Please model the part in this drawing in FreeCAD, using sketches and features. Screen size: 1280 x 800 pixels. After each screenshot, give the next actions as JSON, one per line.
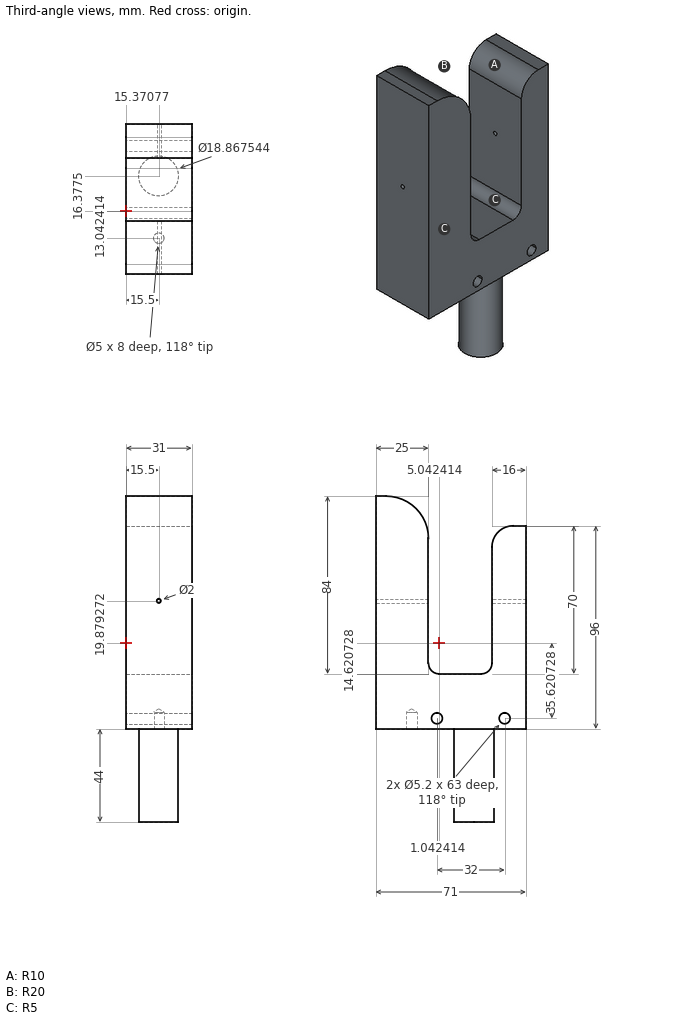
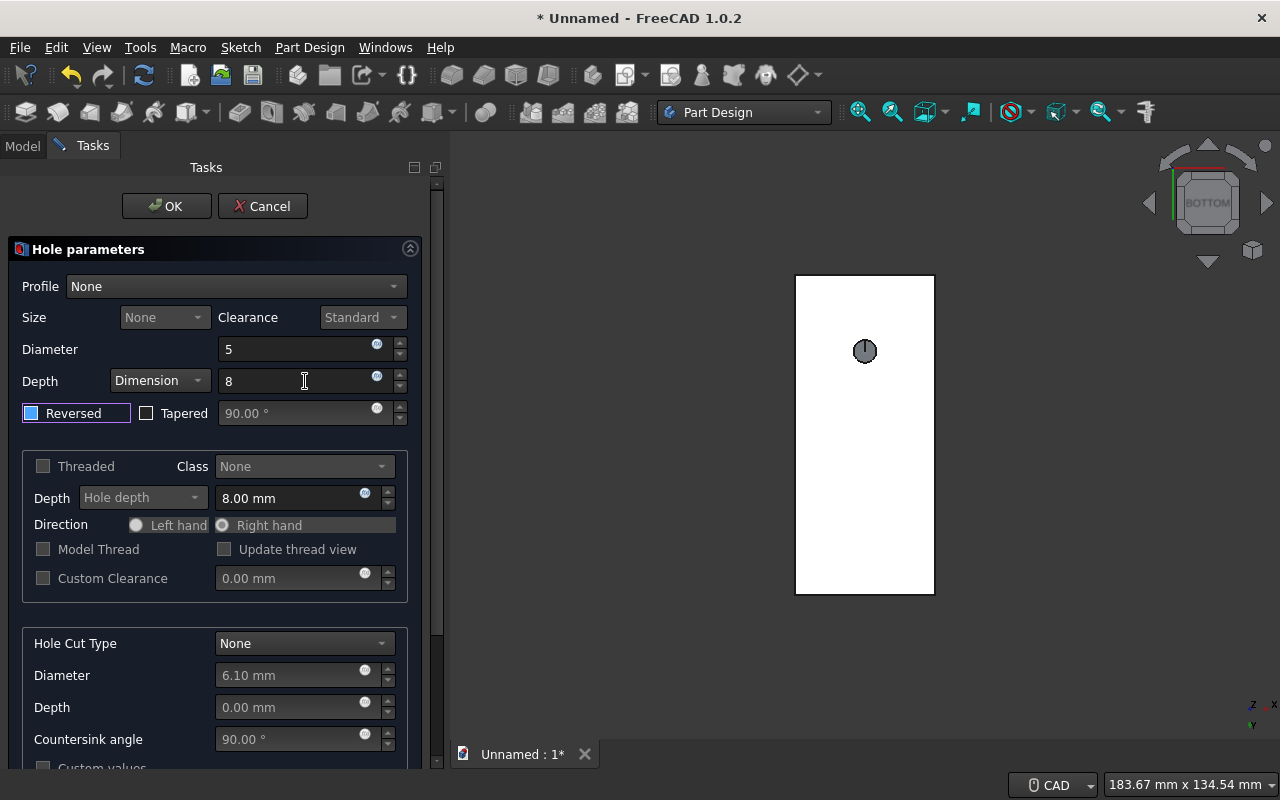
{"action": "left_click", "coordinate": [167, 206]}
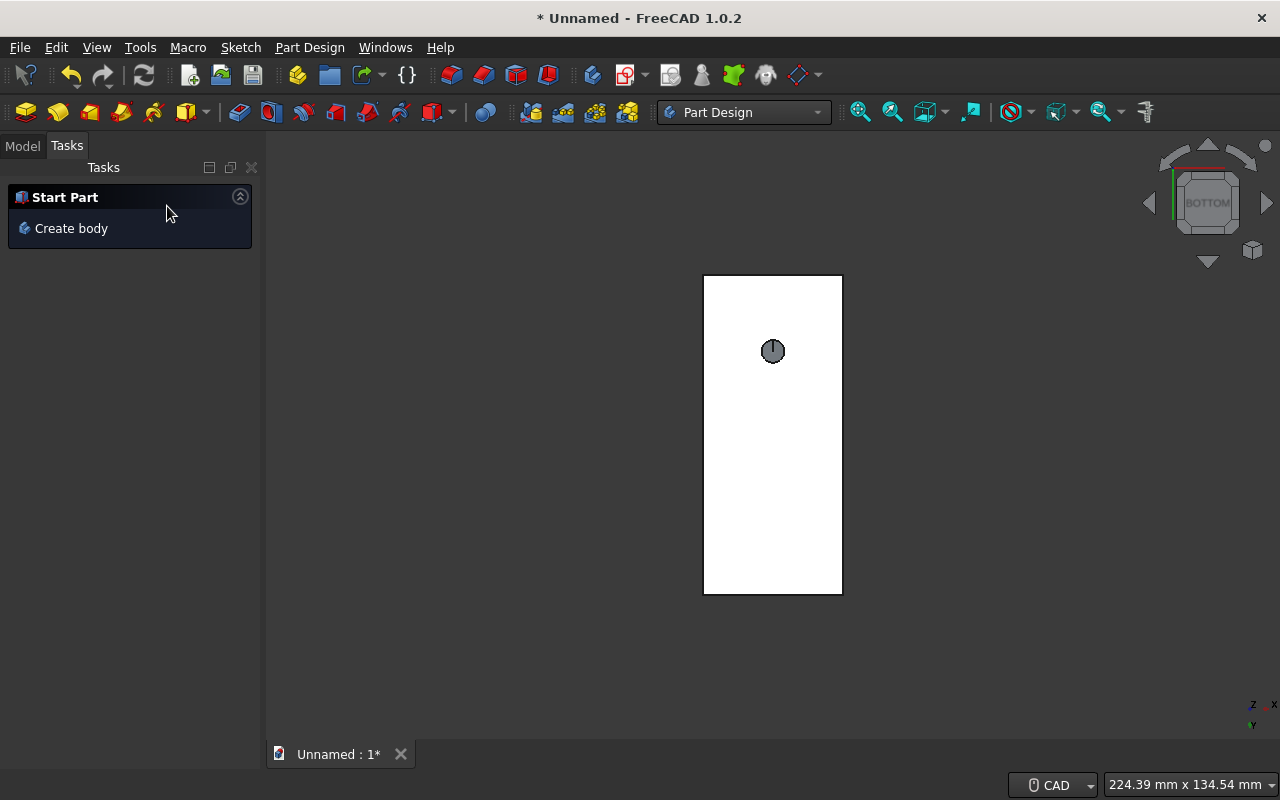
{"action": "left_click", "coordinate": [773, 480]}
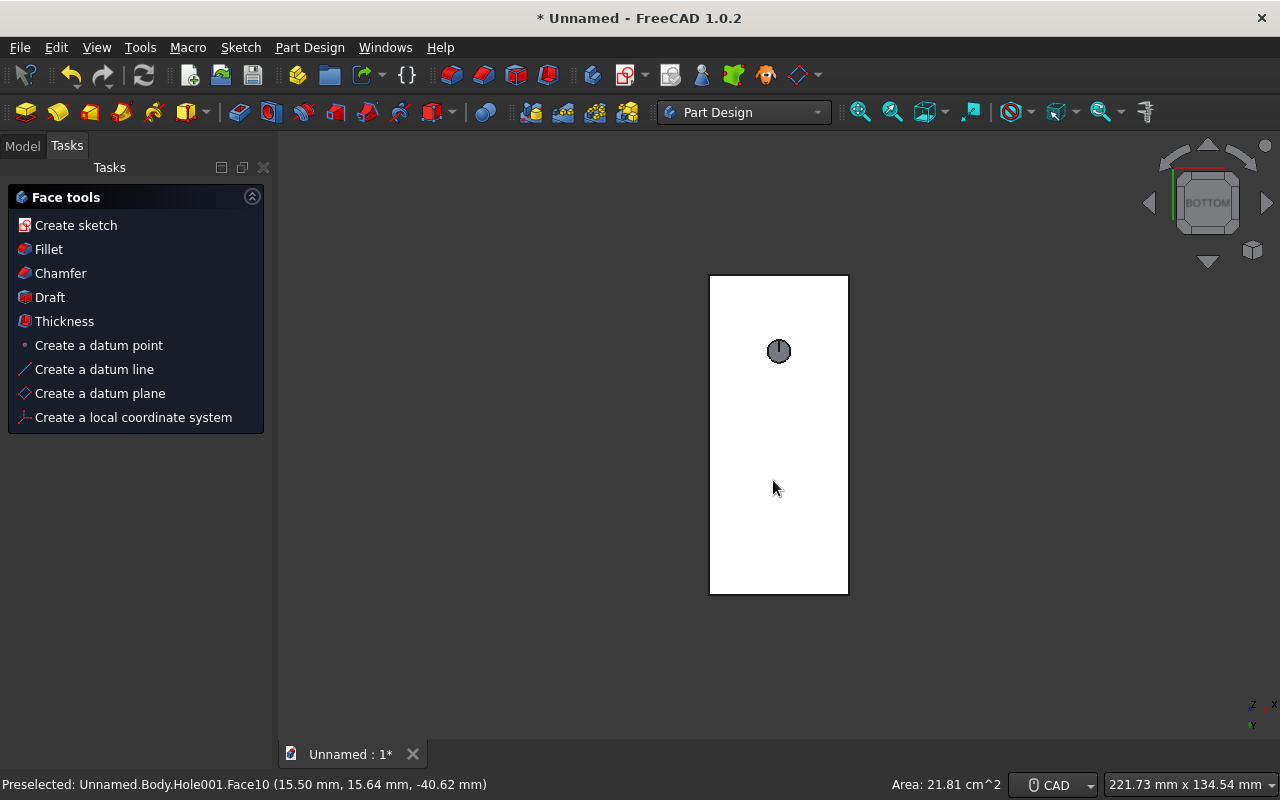
{"action": "left_click", "coordinate": [626, 76]}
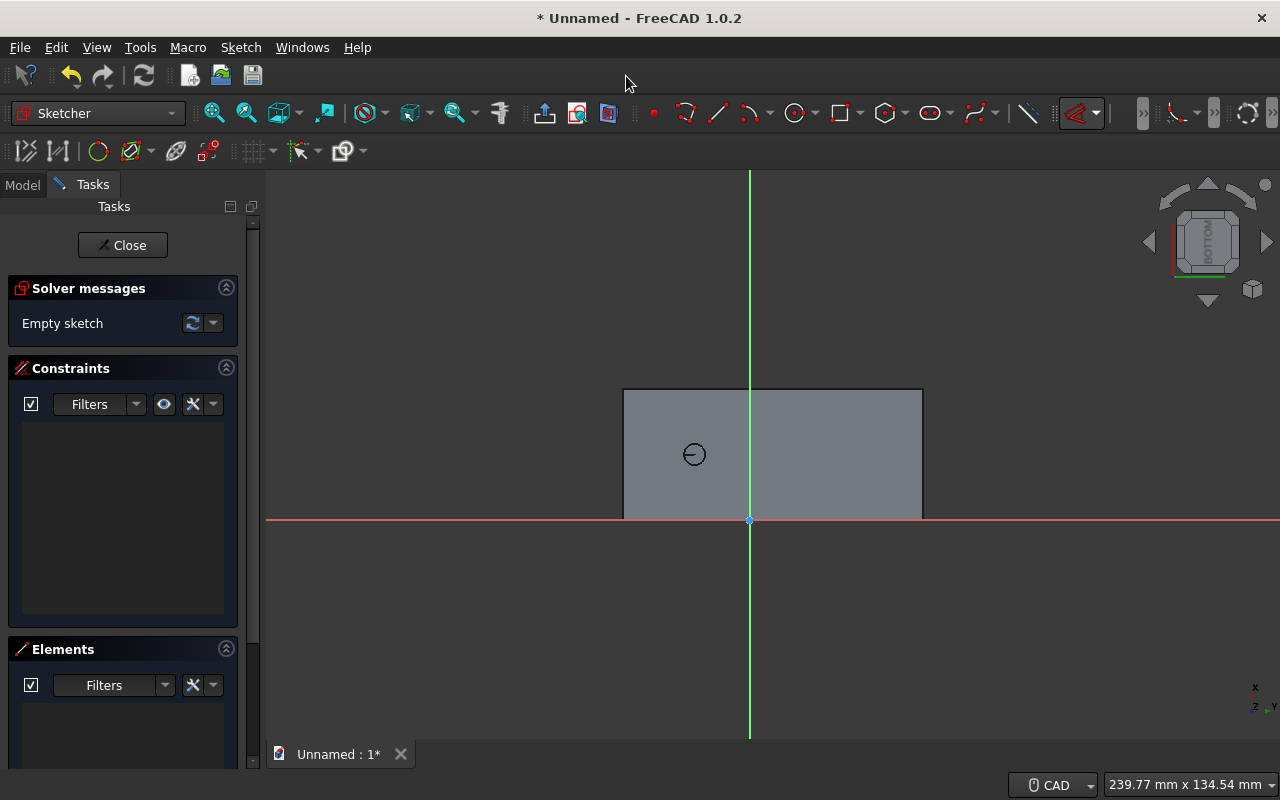
{"action": "scroll", "coordinate": [848, 473], "scroll_direction": "up", "scroll_amount": 6}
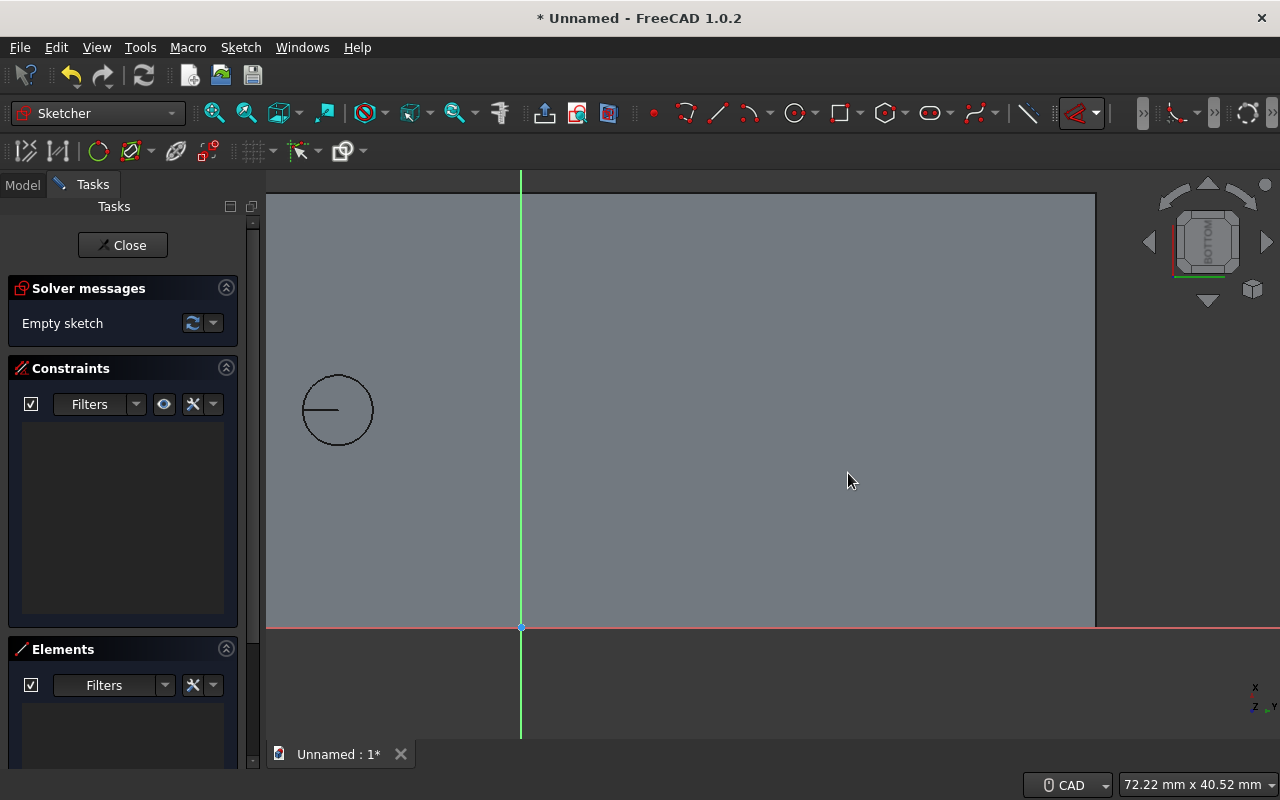
{"action": "left_click", "coordinate": [796, 114]}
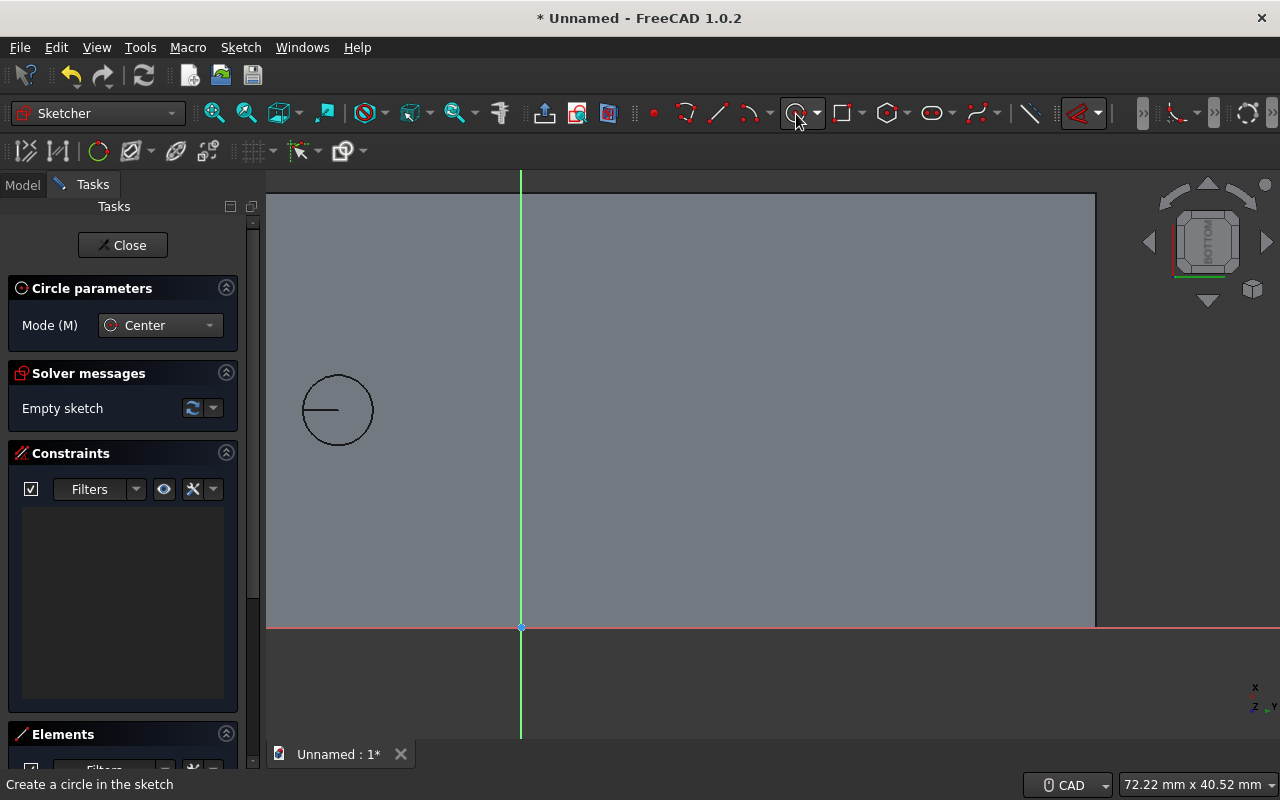
{"action": "left_click", "coordinate": [751, 412]}
{"action": "mouse_move", "coordinate": [845, 318]}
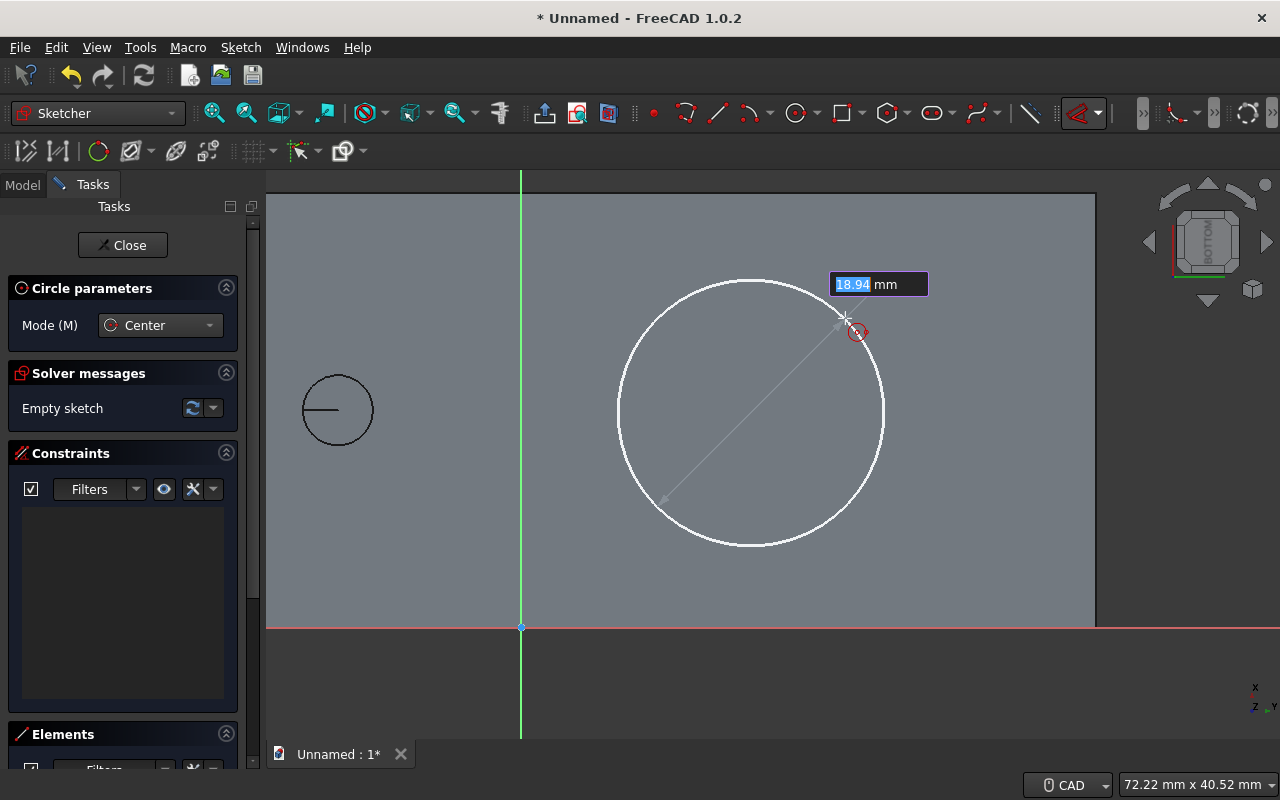
{"action": "type", "text": "18.867544"}
{"action": "key", "text": "Return"}
{"action": "key", "text": "Escape"}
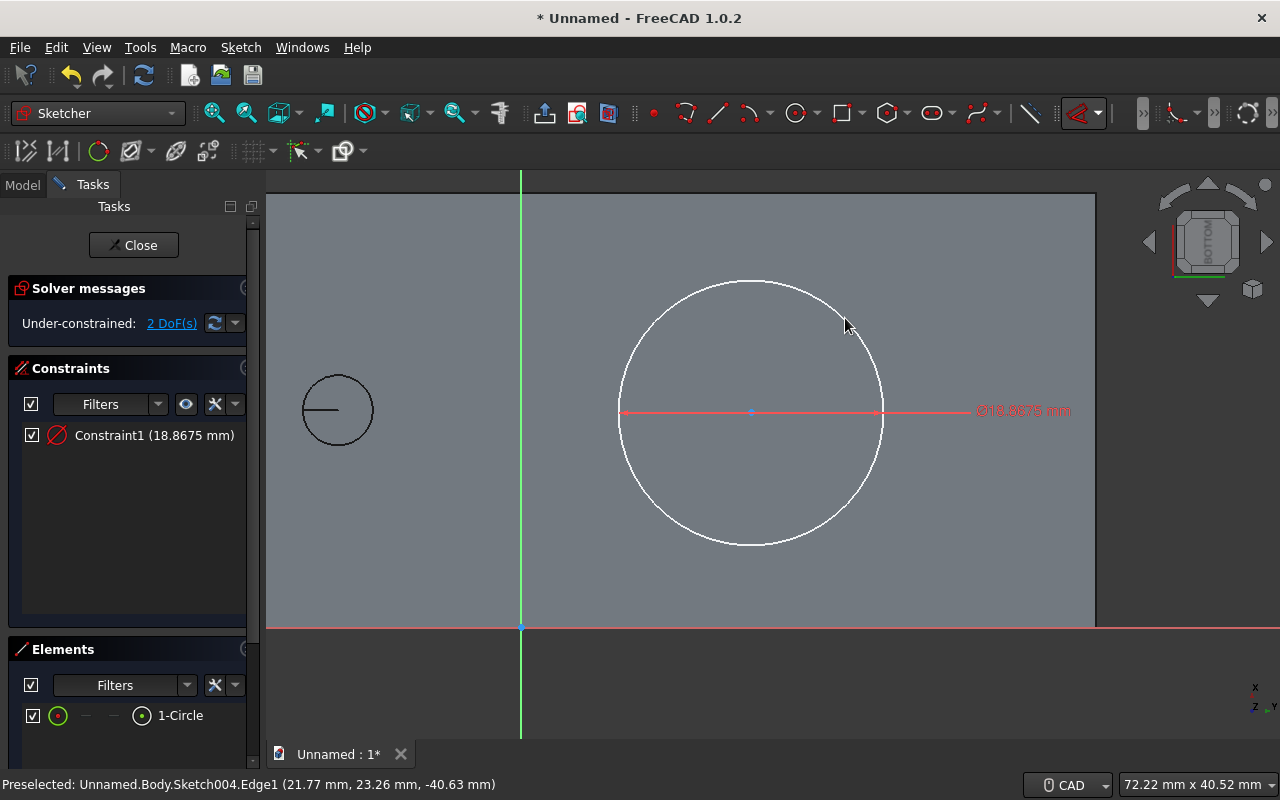
{"action": "left_click", "coordinate": [751, 413]}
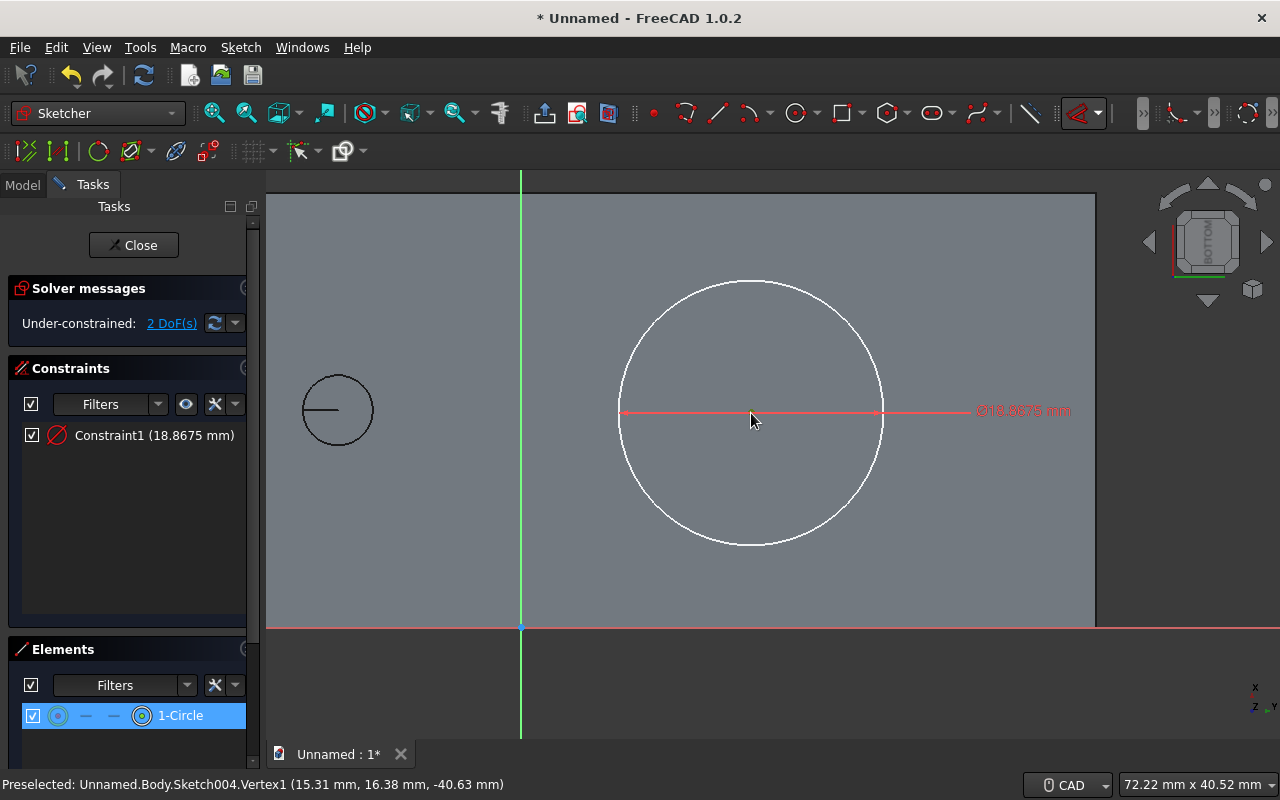
{"action": "key", "text": "l"}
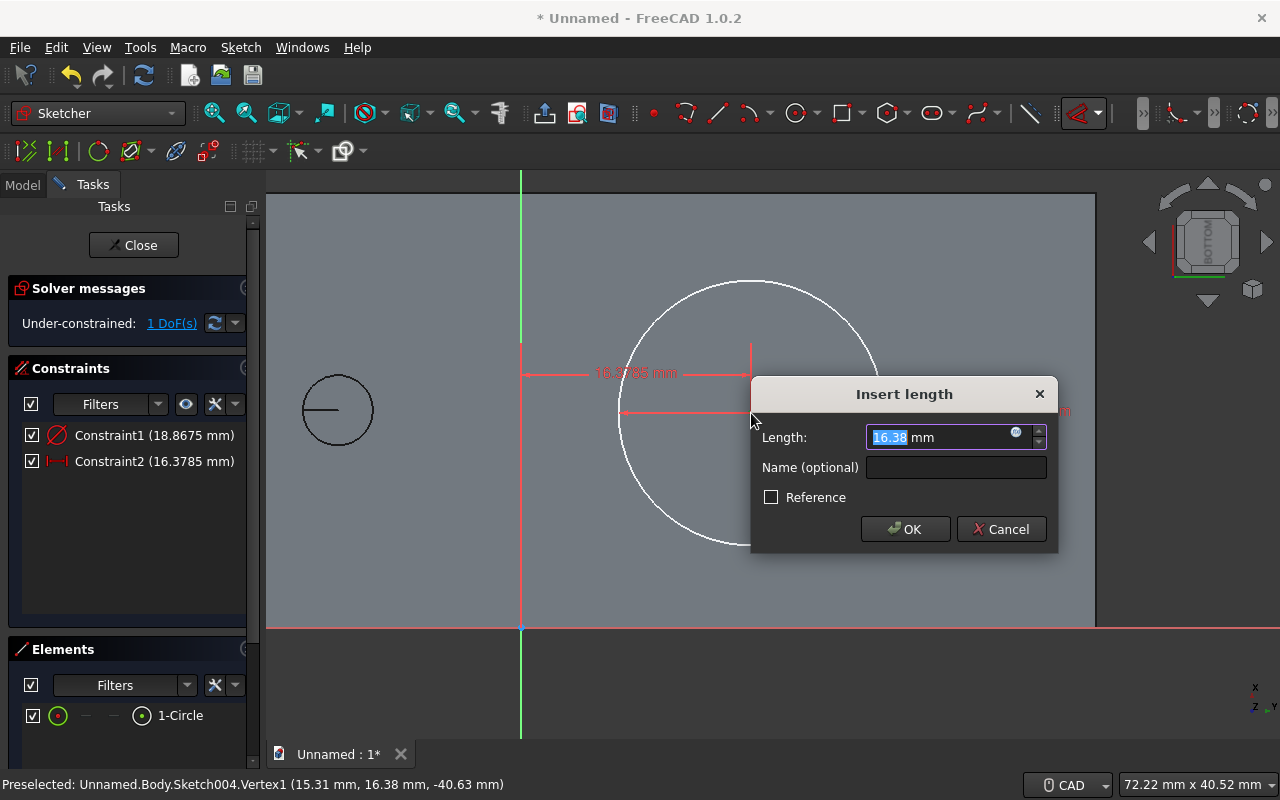
{"action": "type", "text": "16.3775"}
{"action": "key", "text": "Return"}